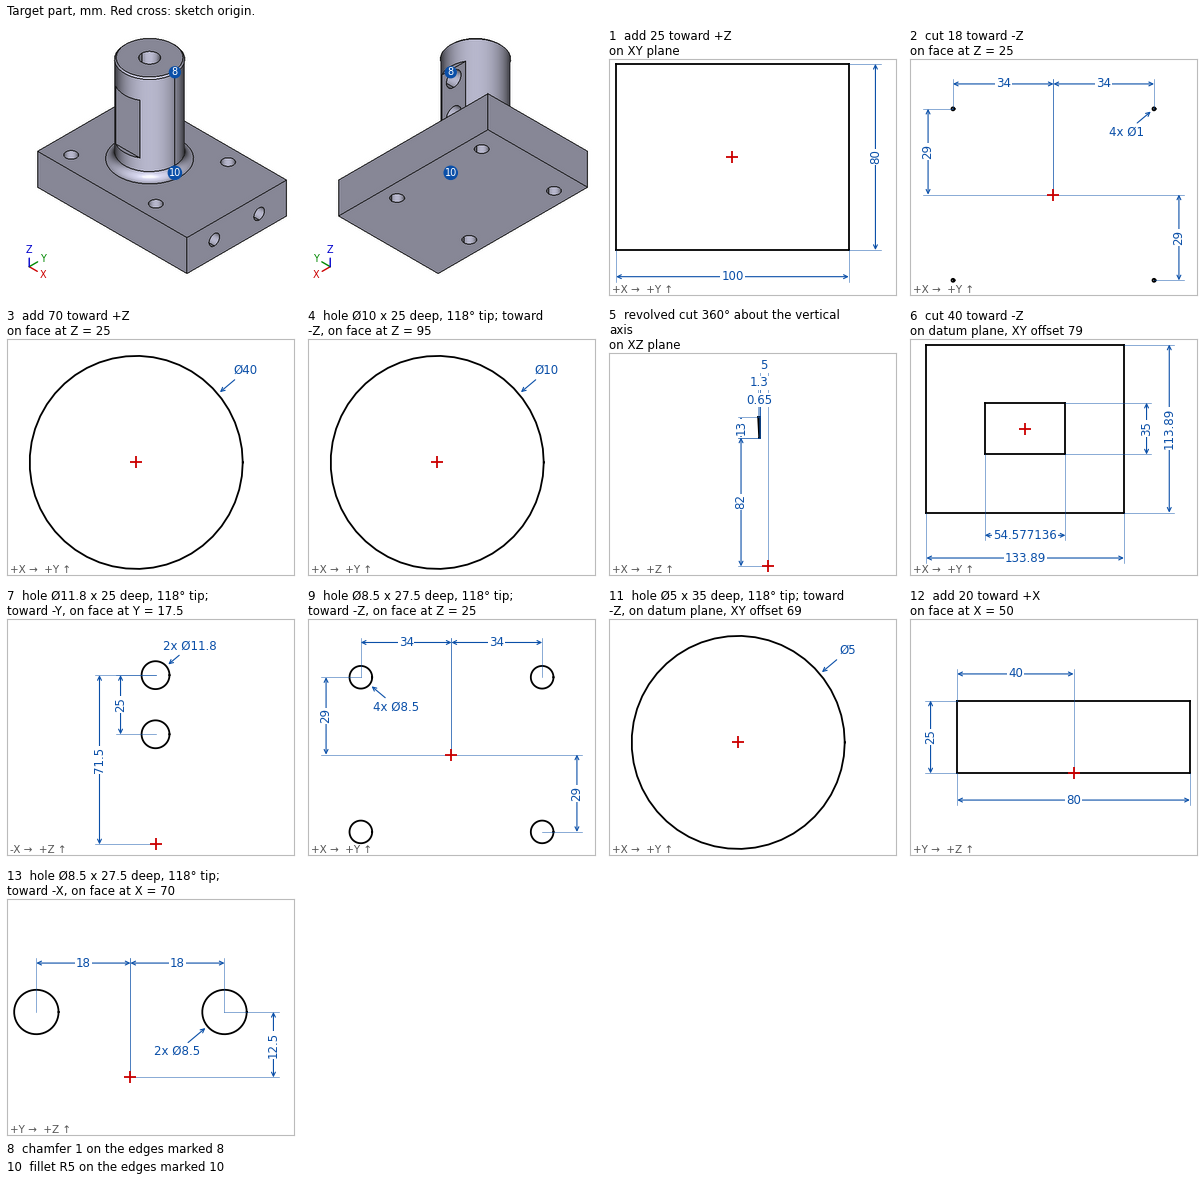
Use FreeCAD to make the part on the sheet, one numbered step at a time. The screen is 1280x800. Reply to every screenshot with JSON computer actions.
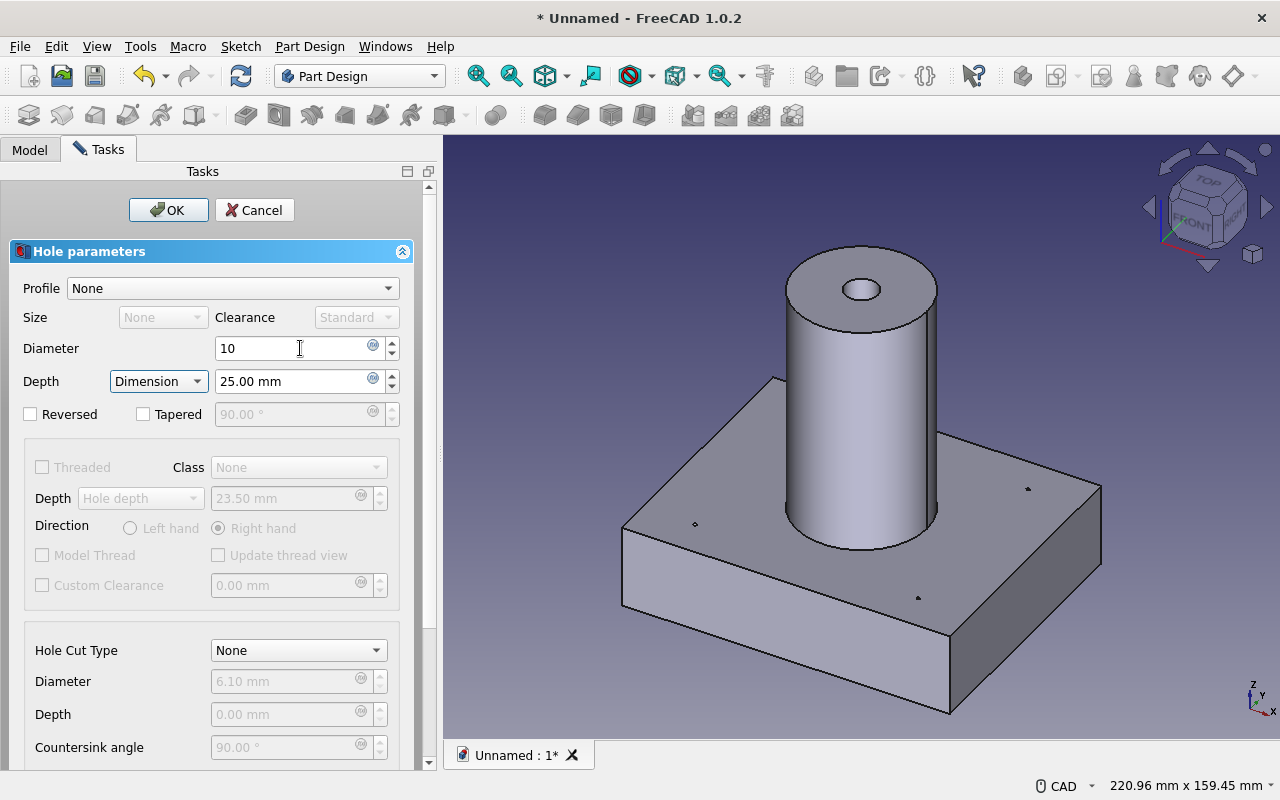
{"action": "triple_click", "coordinate": [300, 382]}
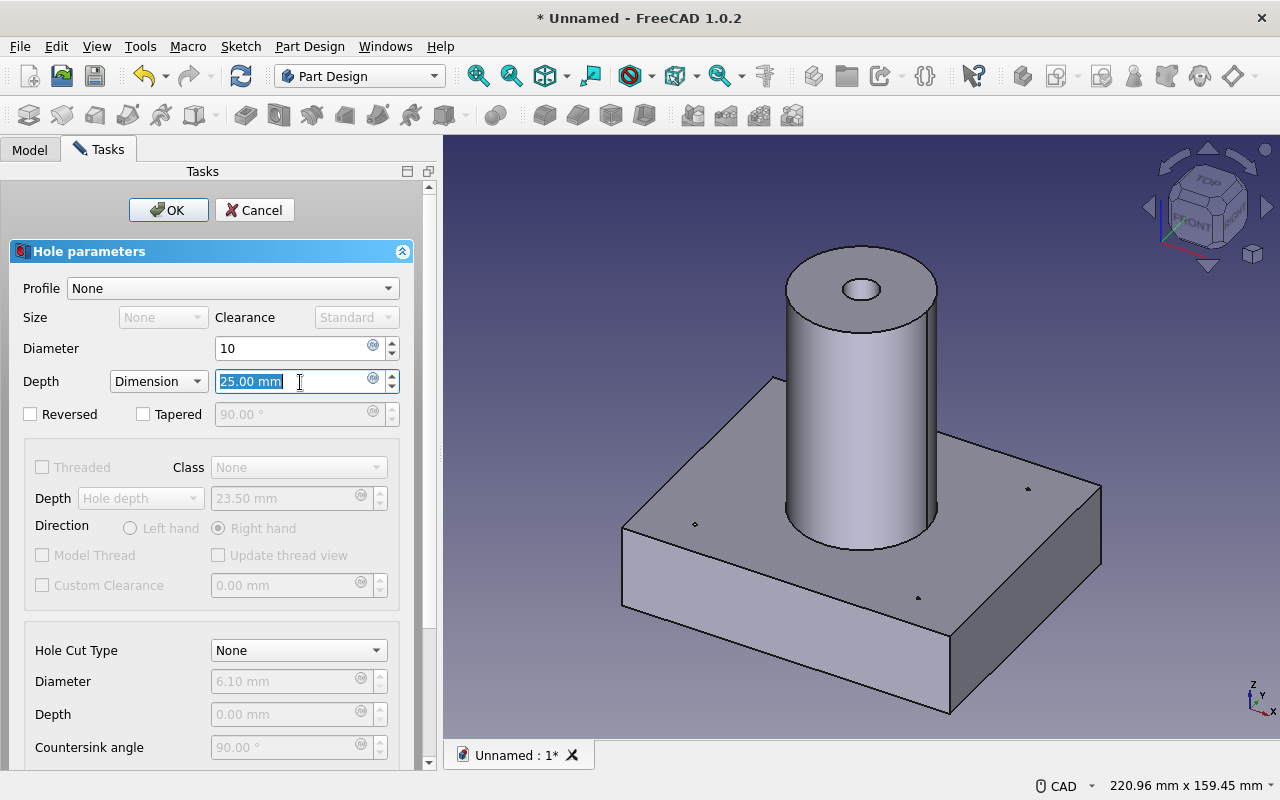
{"action": "type", "text": "25"}
{"action": "key", "text": "Tab"}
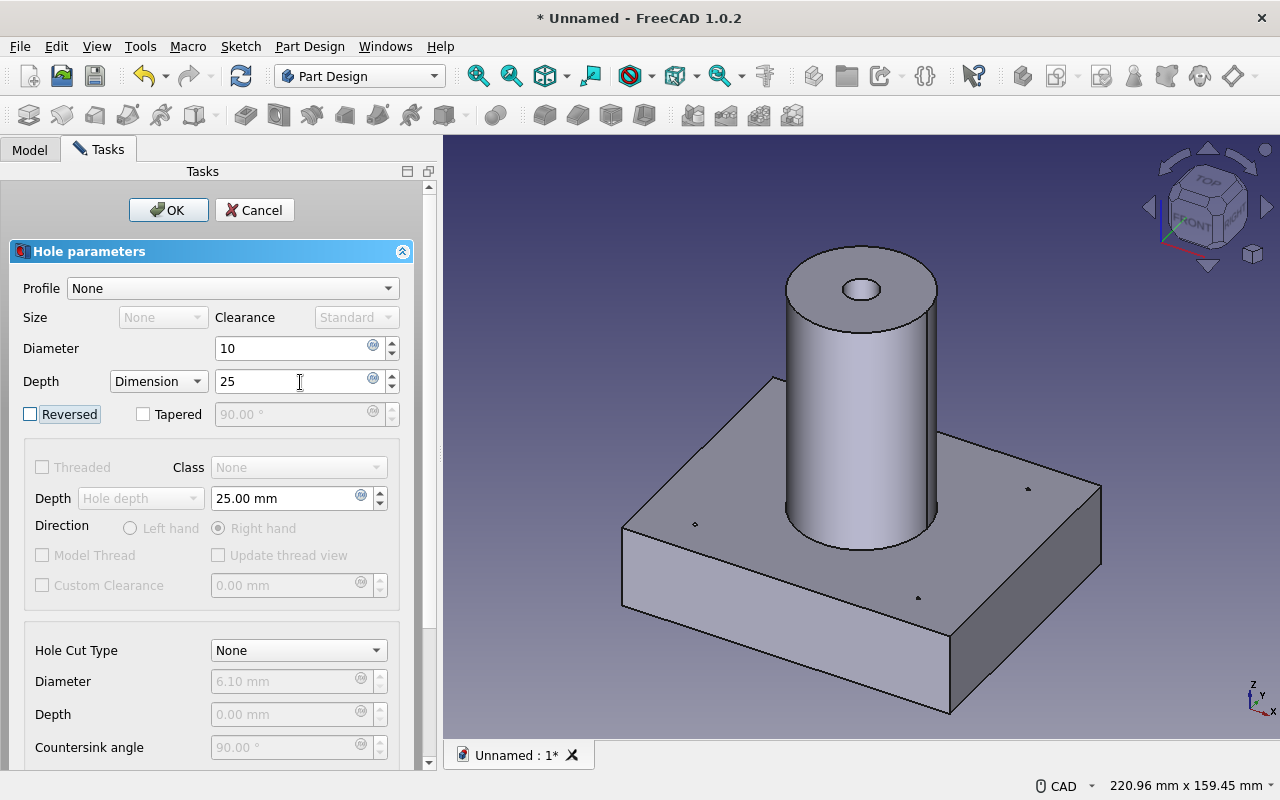
{"action": "left_click", "coordinate": [169, 210]}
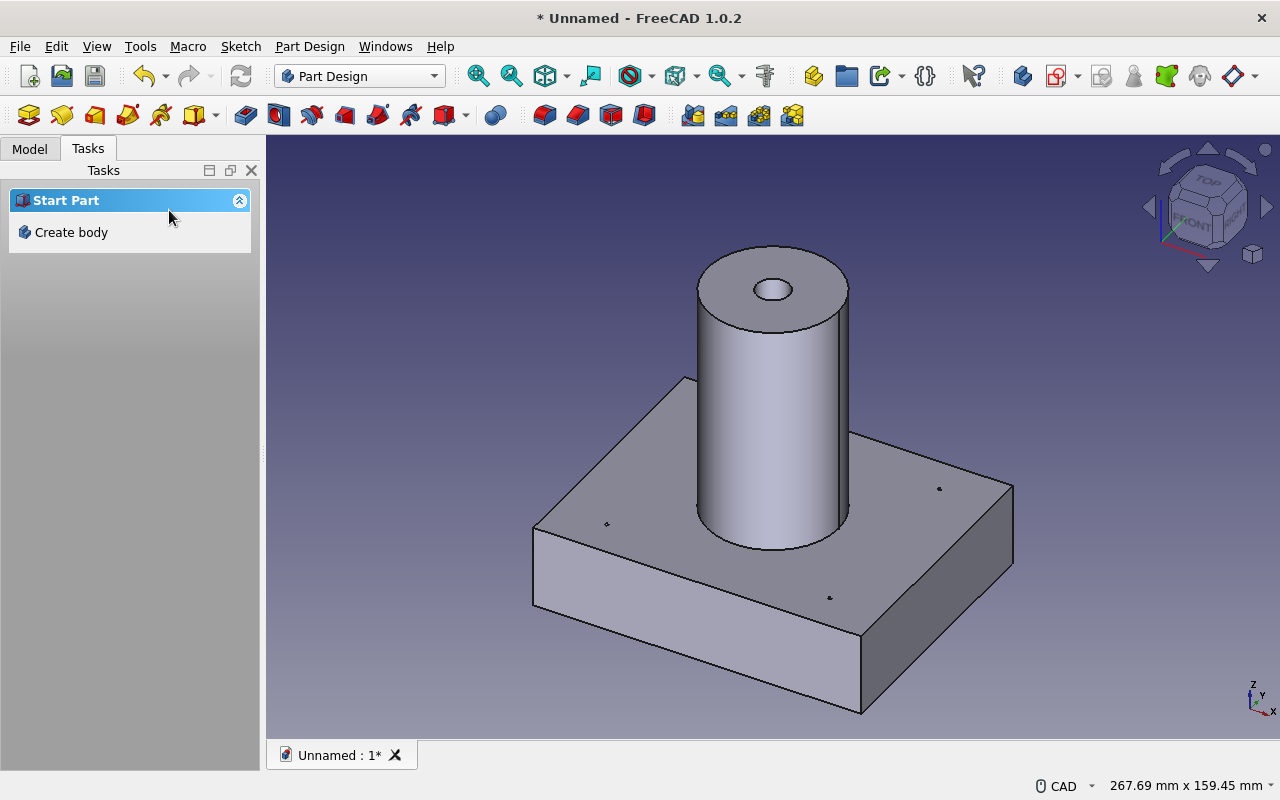
{"action": "left_click", "coordinate": [1056, 76]}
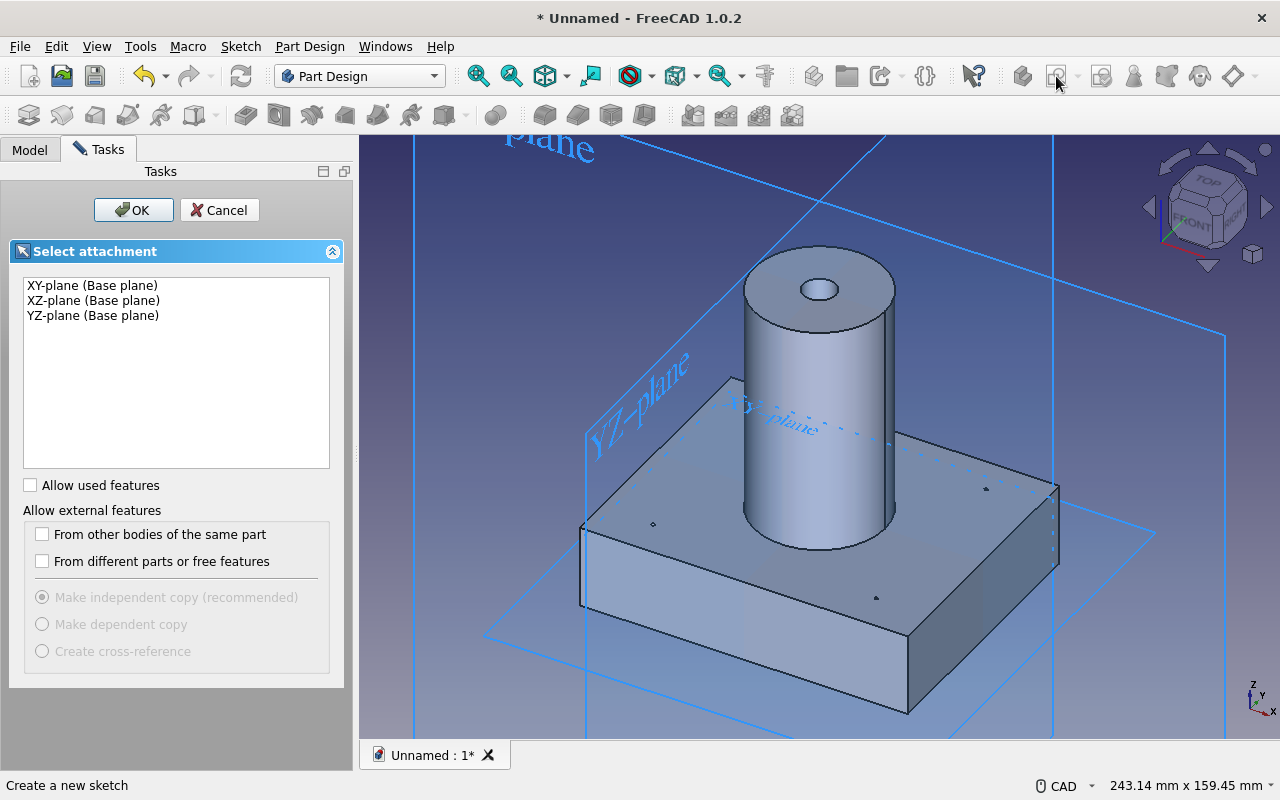
{"action": "left_click", "coordinate": [84, 300]}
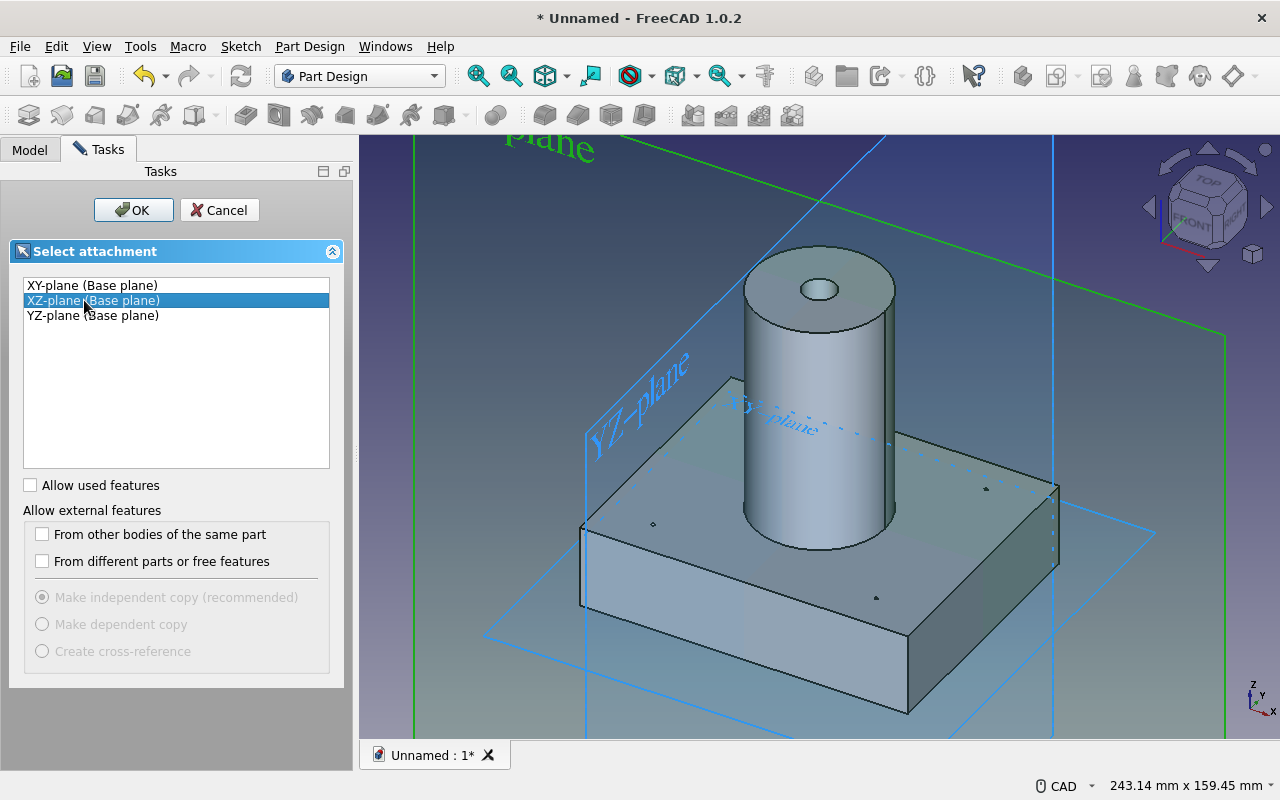
{"action": "left_click", "coordinate": [134, 210]}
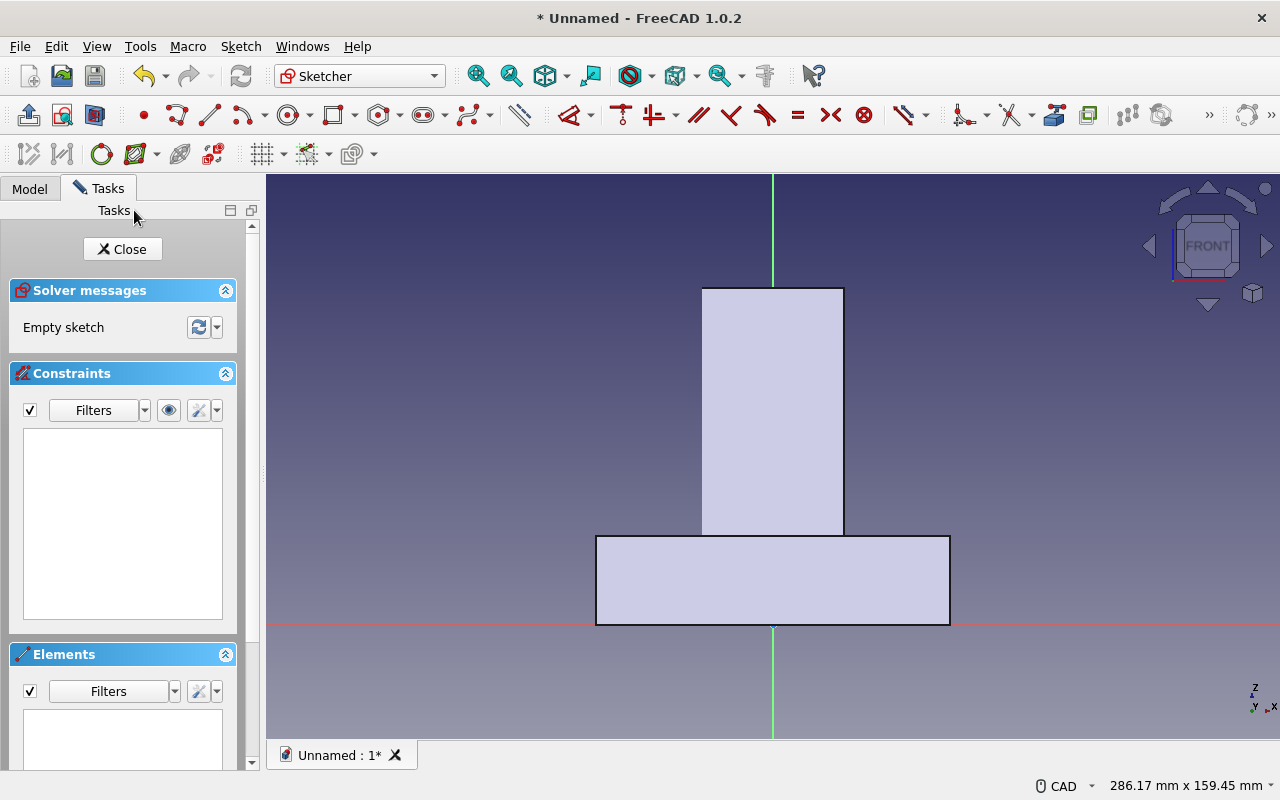
{"action": "left_click", "coordinate": [95, 116]}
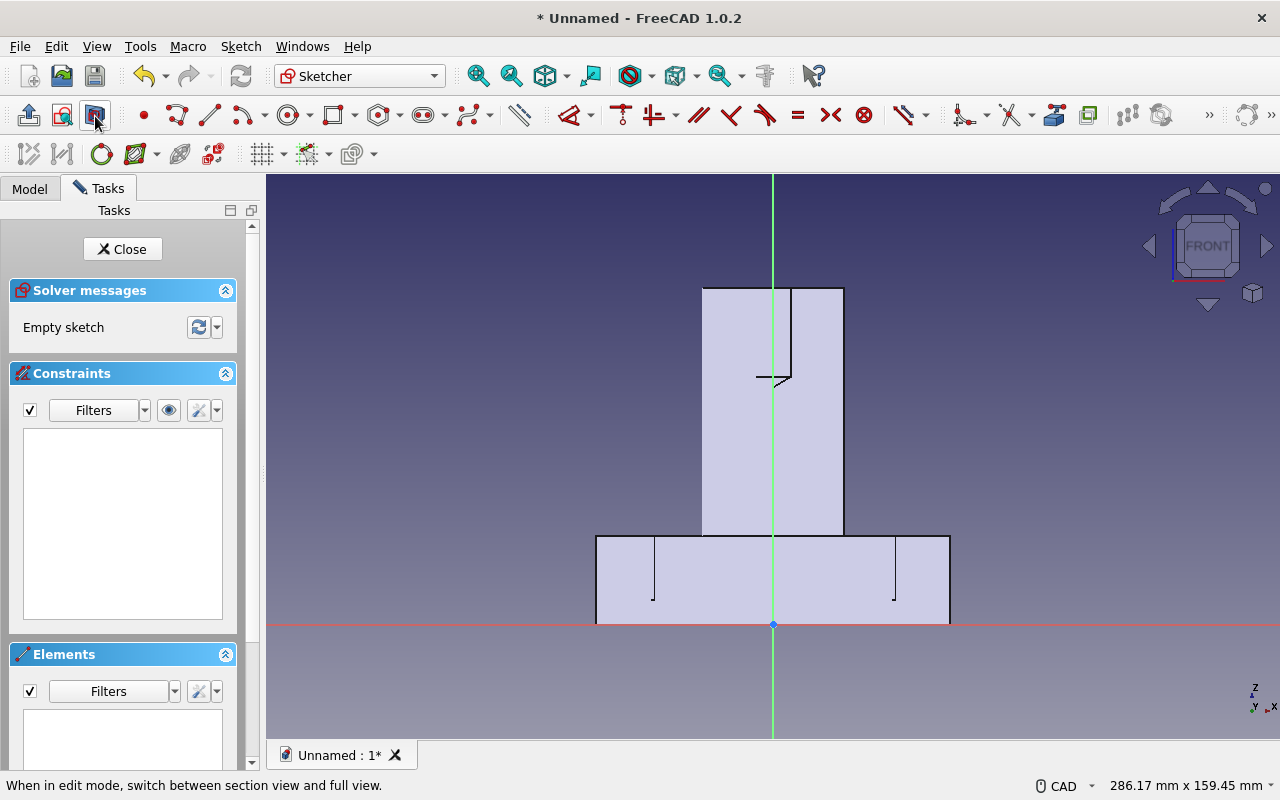
{"action": "scroll", "coordinate": [761, 288], "scroll_direction": "up", "scroll_amount": 10}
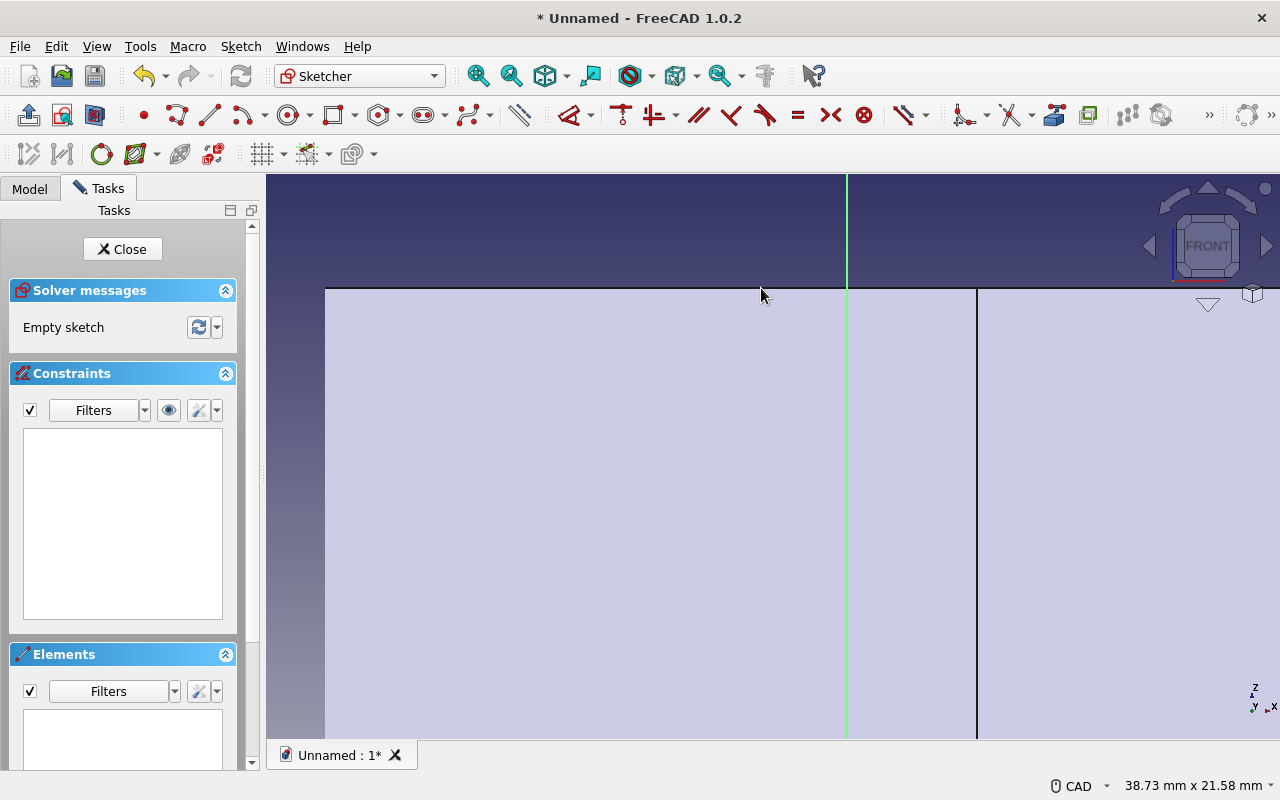
{"action": "key", "text": "g m"}